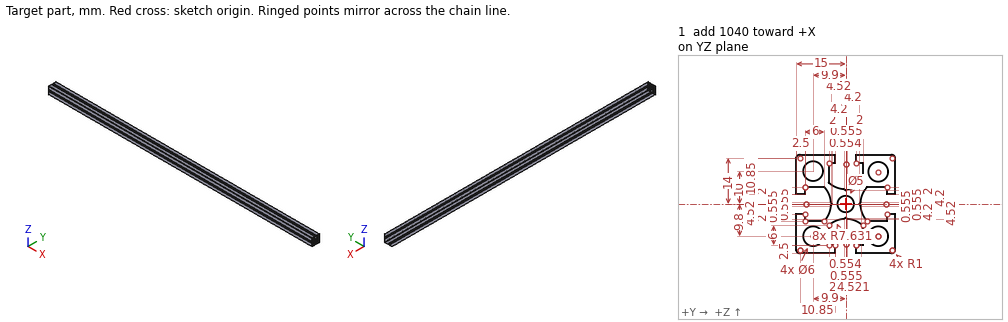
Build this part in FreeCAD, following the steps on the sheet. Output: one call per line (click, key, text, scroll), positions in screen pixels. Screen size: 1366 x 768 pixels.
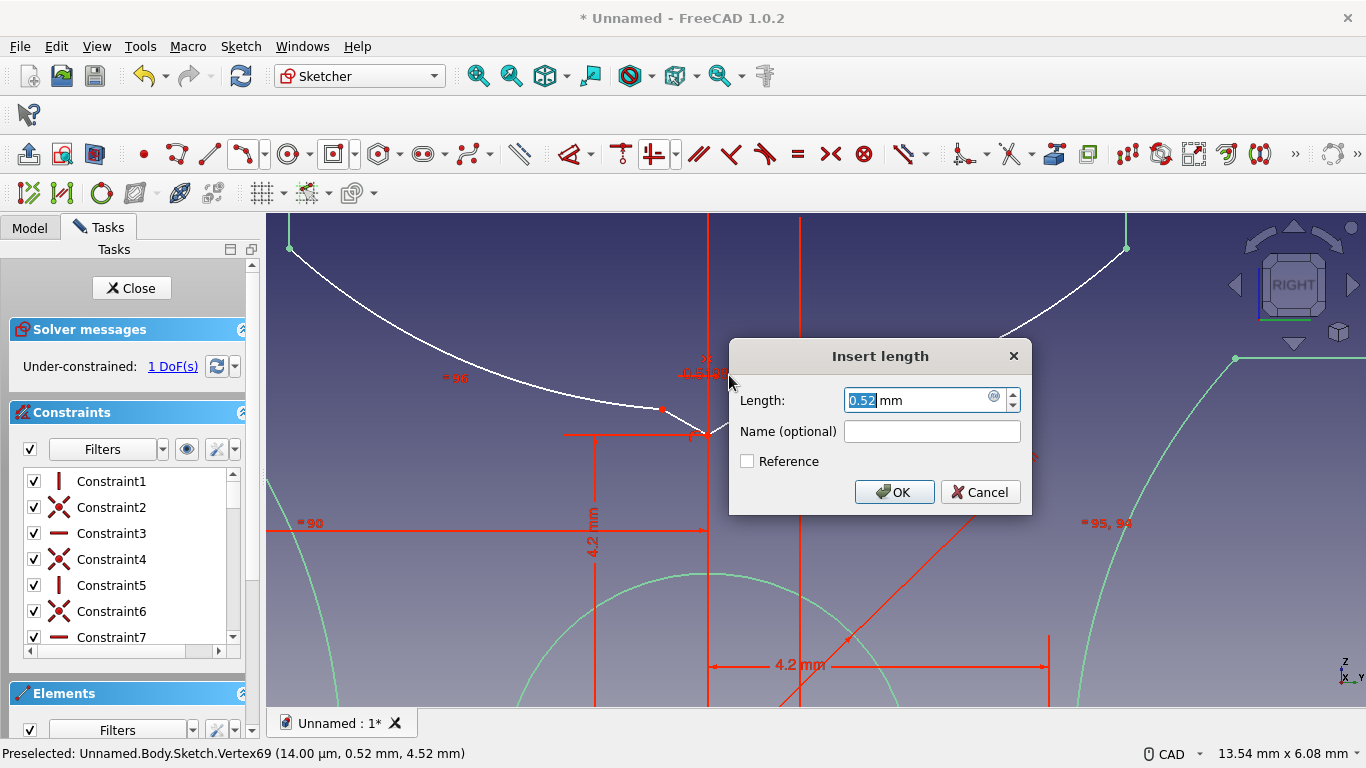
text(0.555)
key(Return)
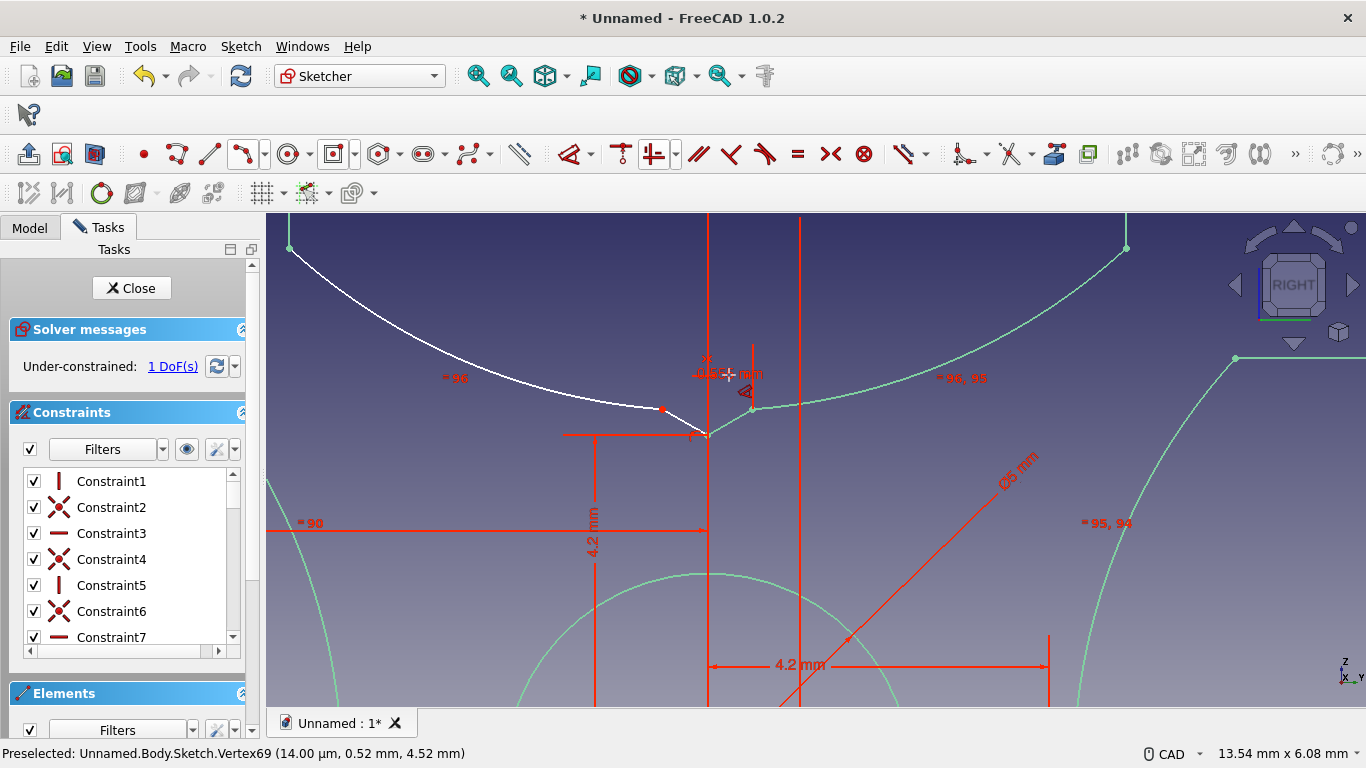
click(662, 409)
click(685, 351)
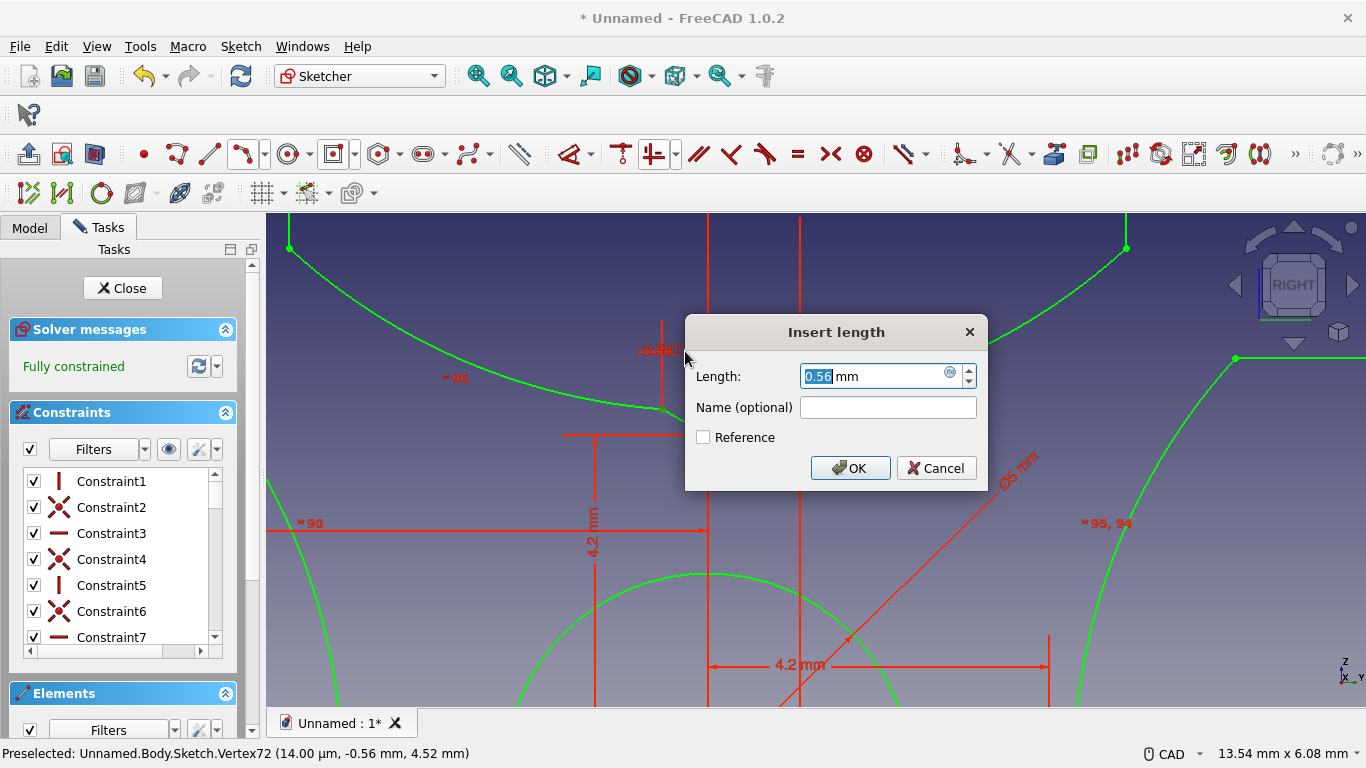
text(0.554)
key(Return)
key(Escape)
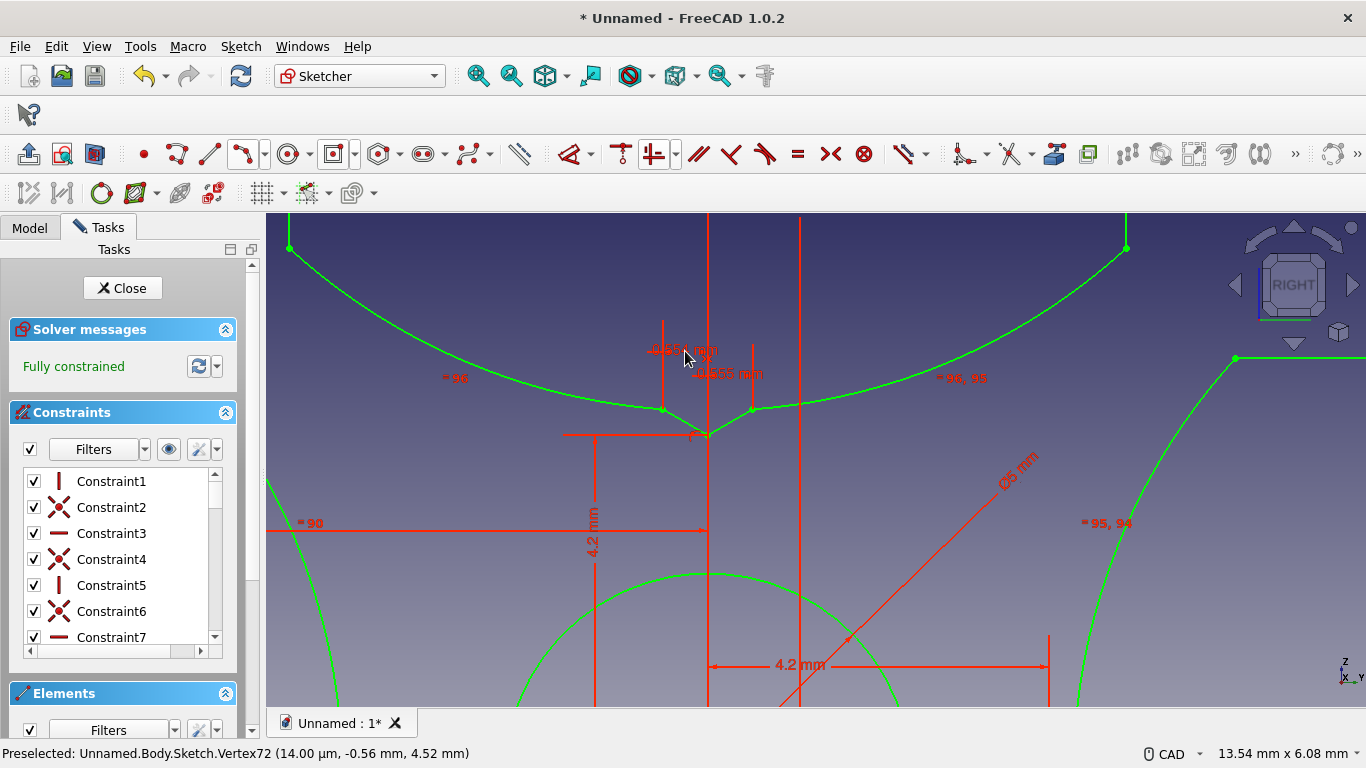
click(123, 288)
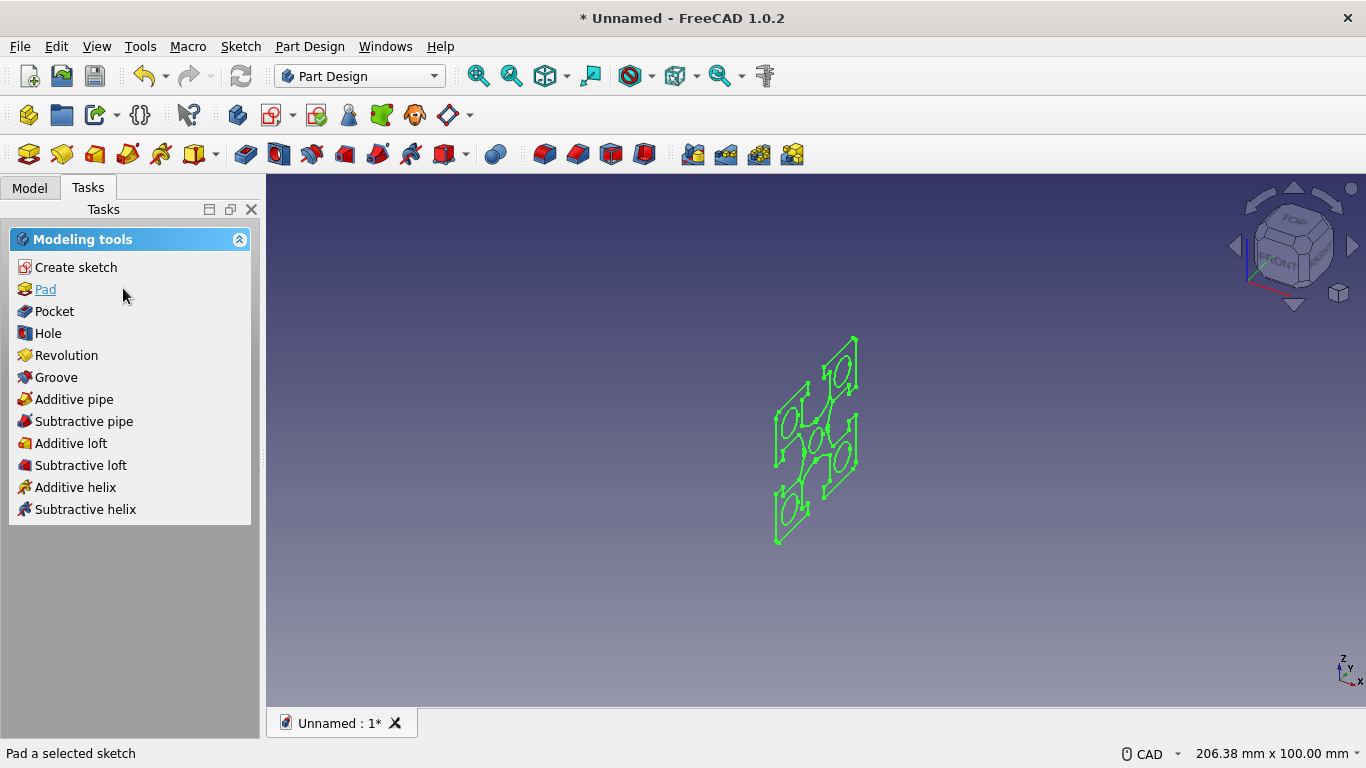
click(29, 154)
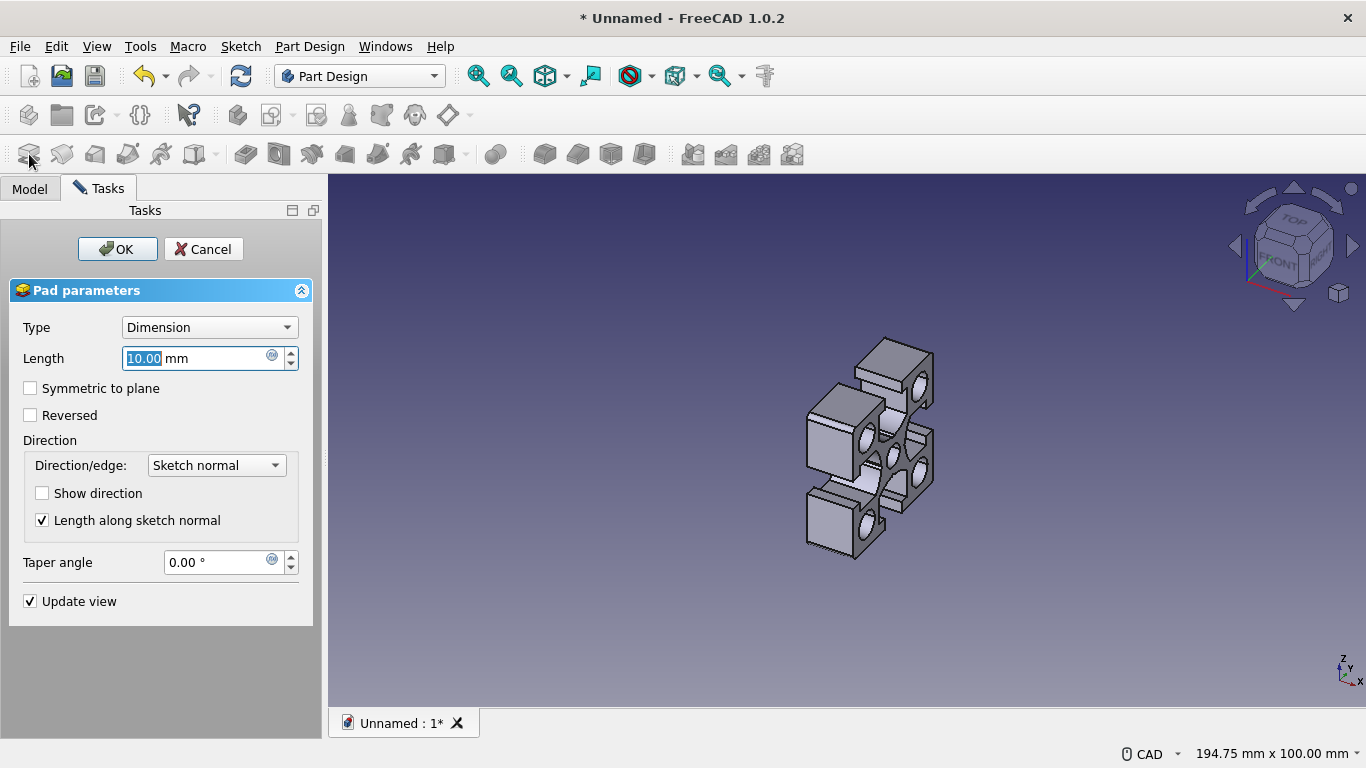
text(1040)
key(Tab)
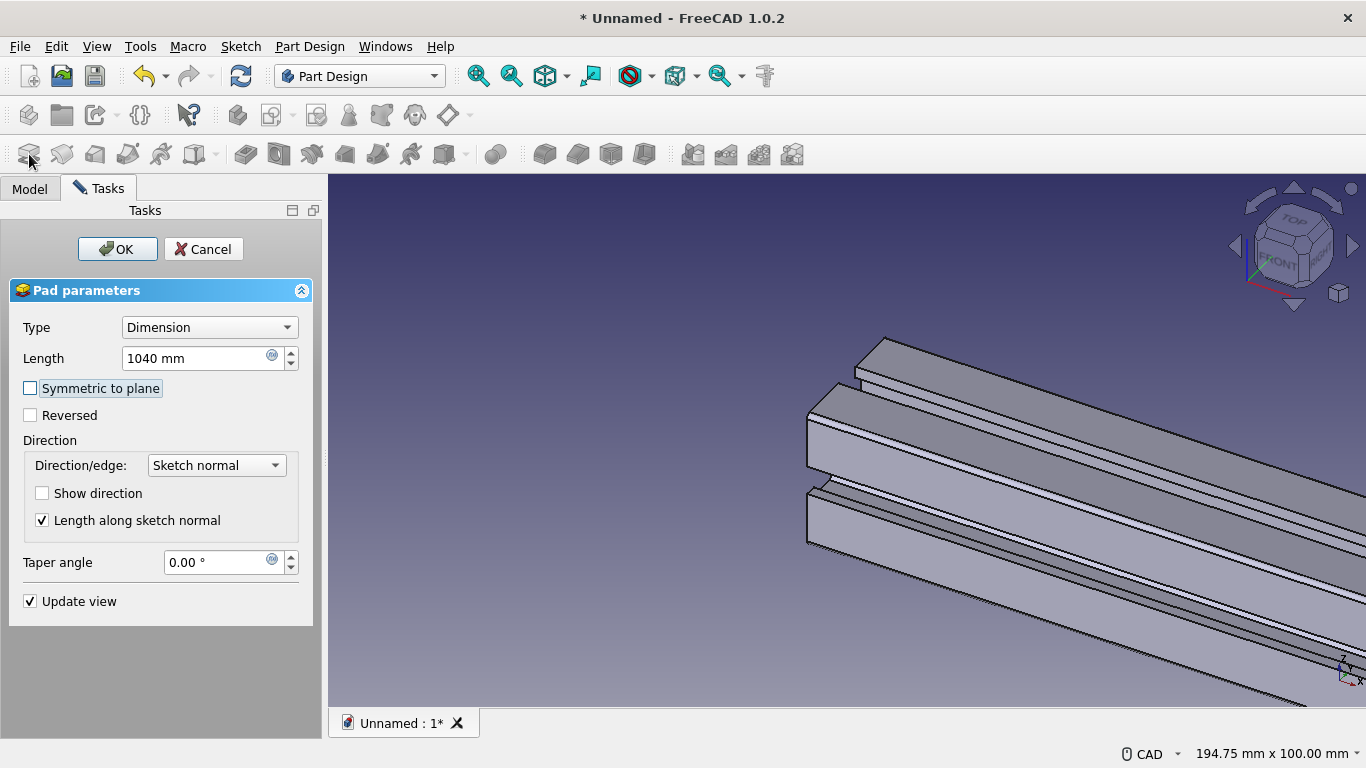
click(118, 249)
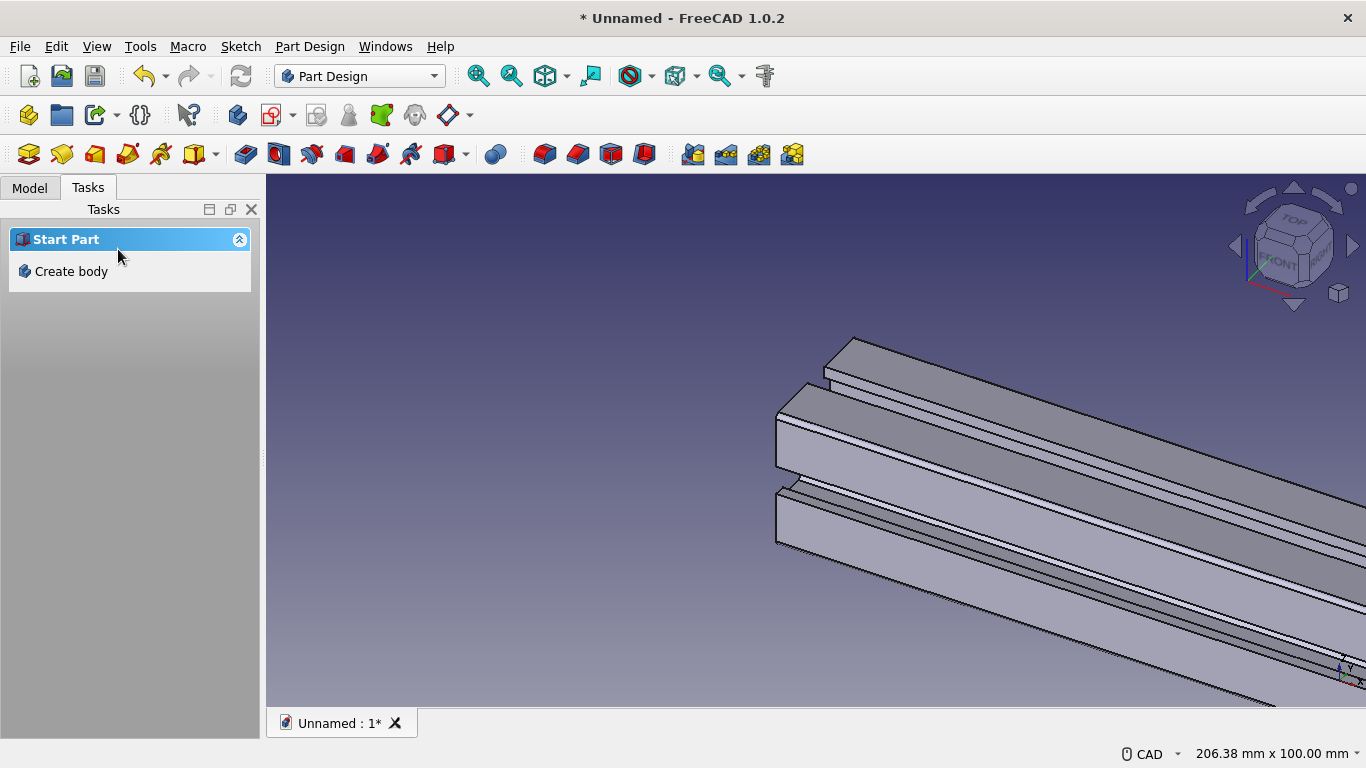
key(0)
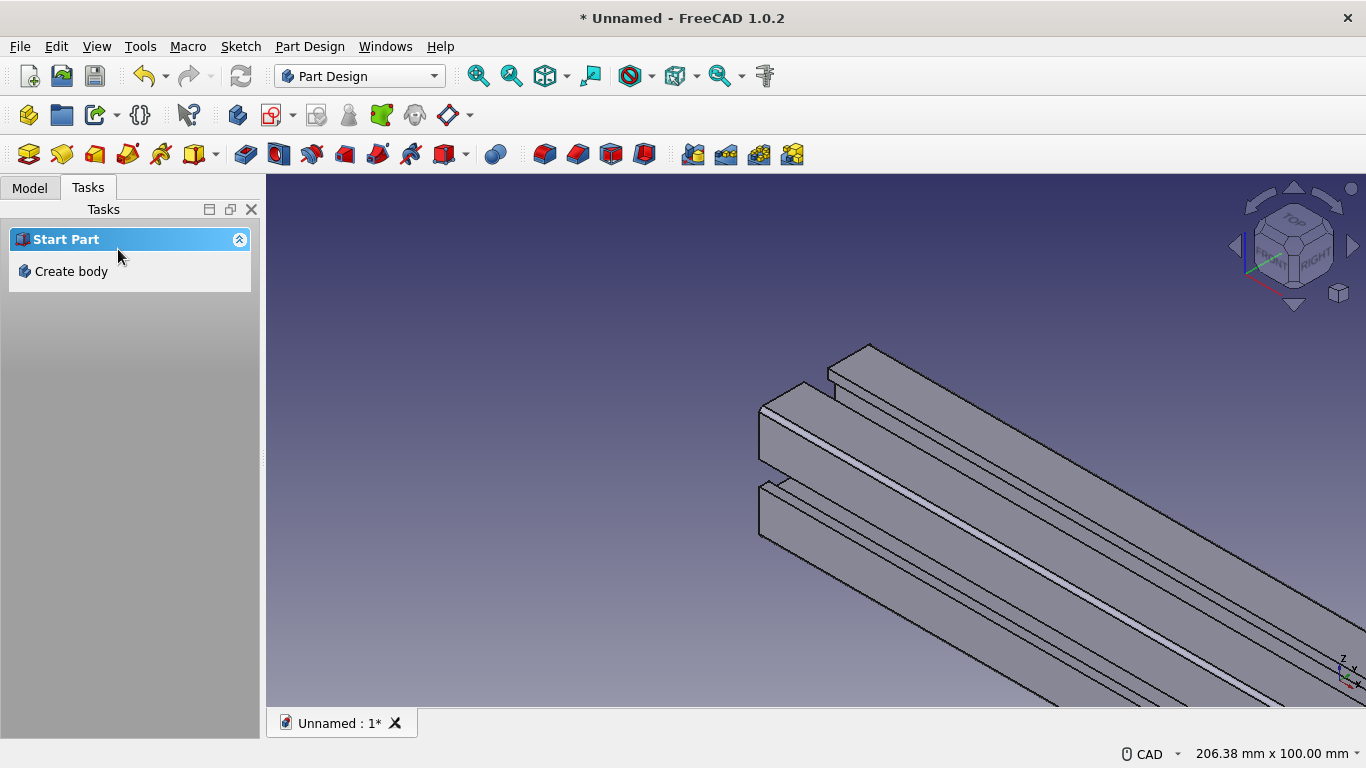
key(v)
key(f)